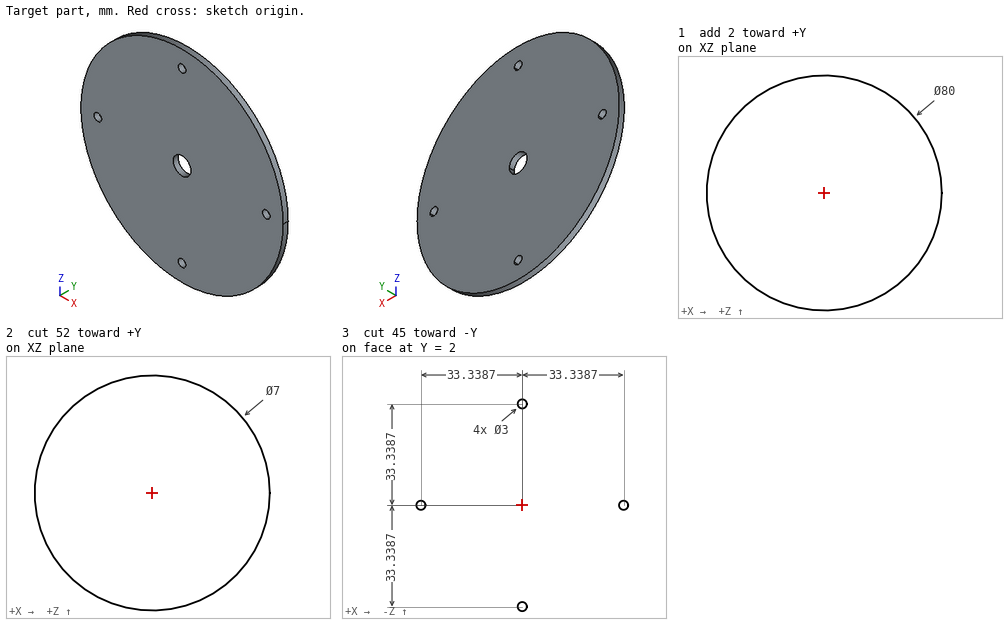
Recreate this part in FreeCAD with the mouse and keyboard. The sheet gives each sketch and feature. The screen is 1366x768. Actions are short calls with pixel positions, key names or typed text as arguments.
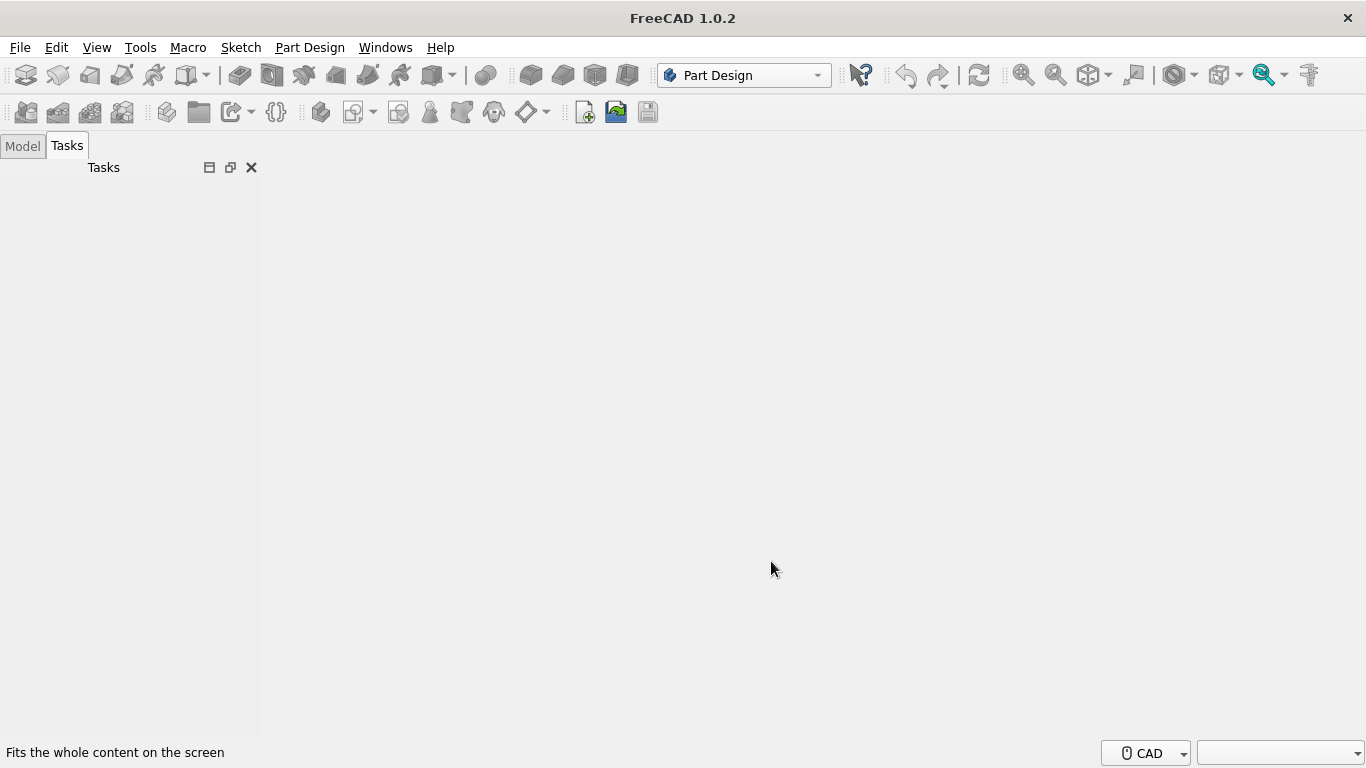
key(ctrl+n)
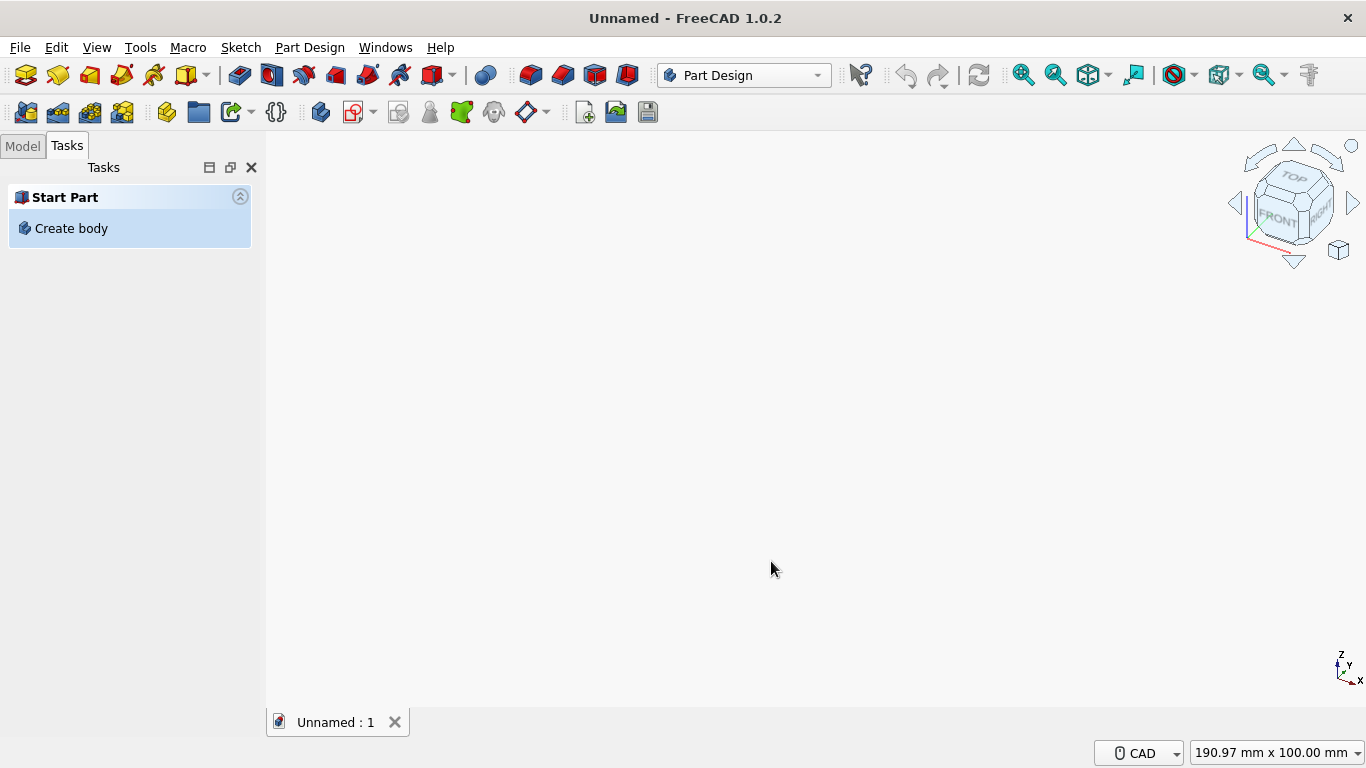
click(354, 112)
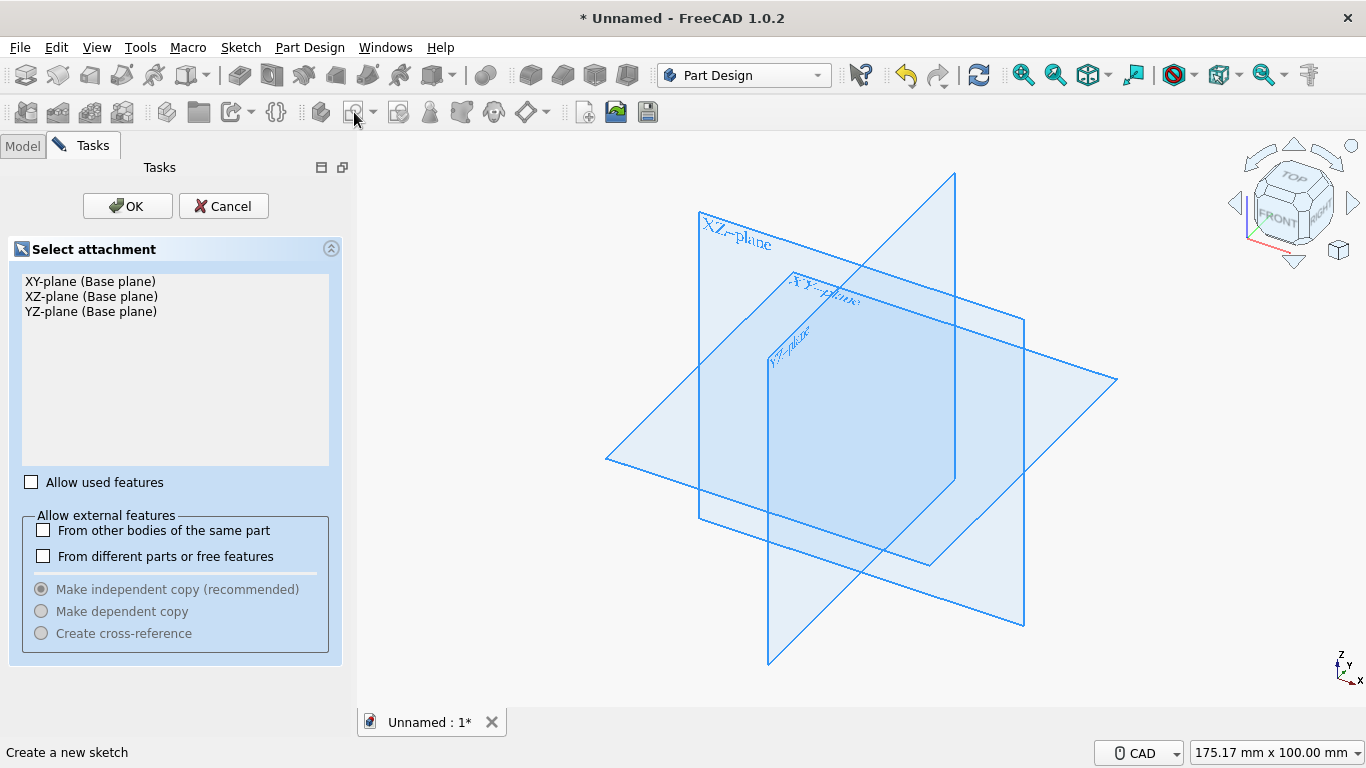
click(82, 296)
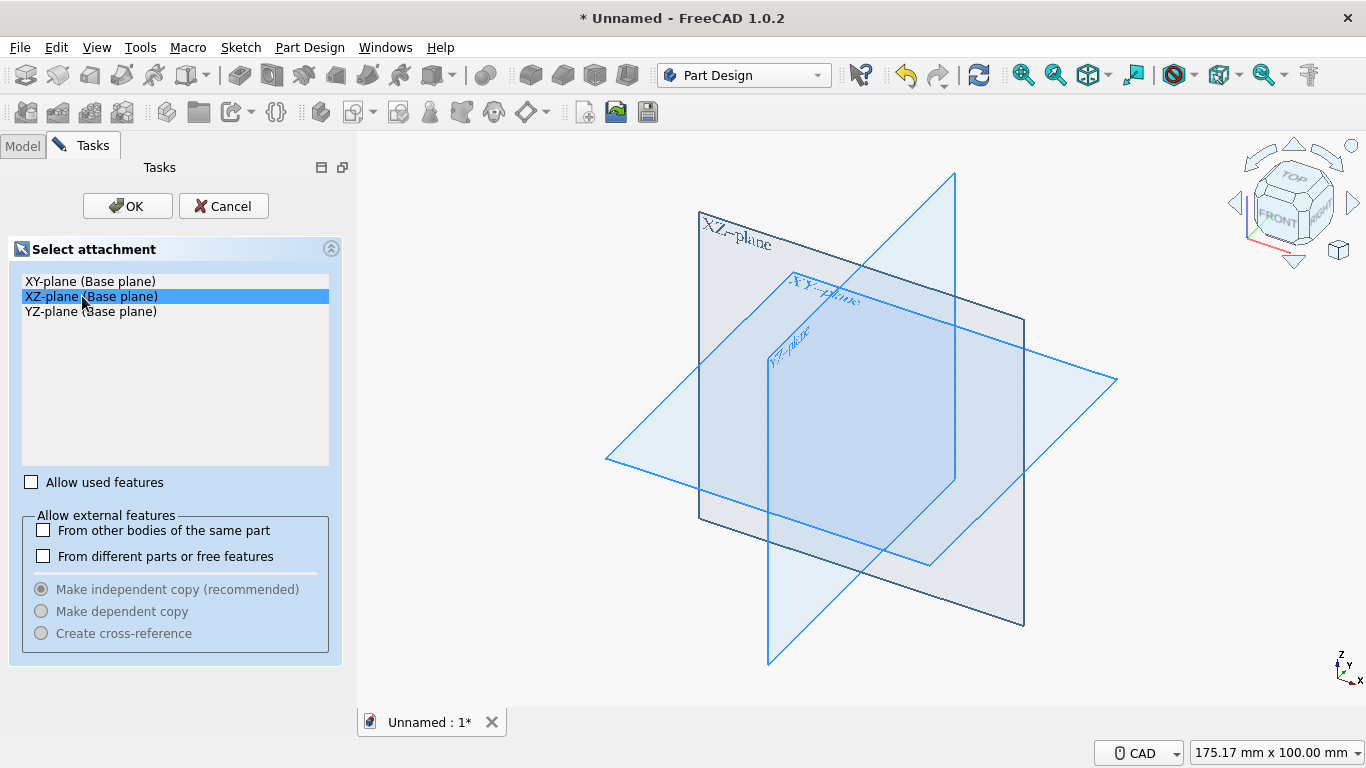
click(128, 206)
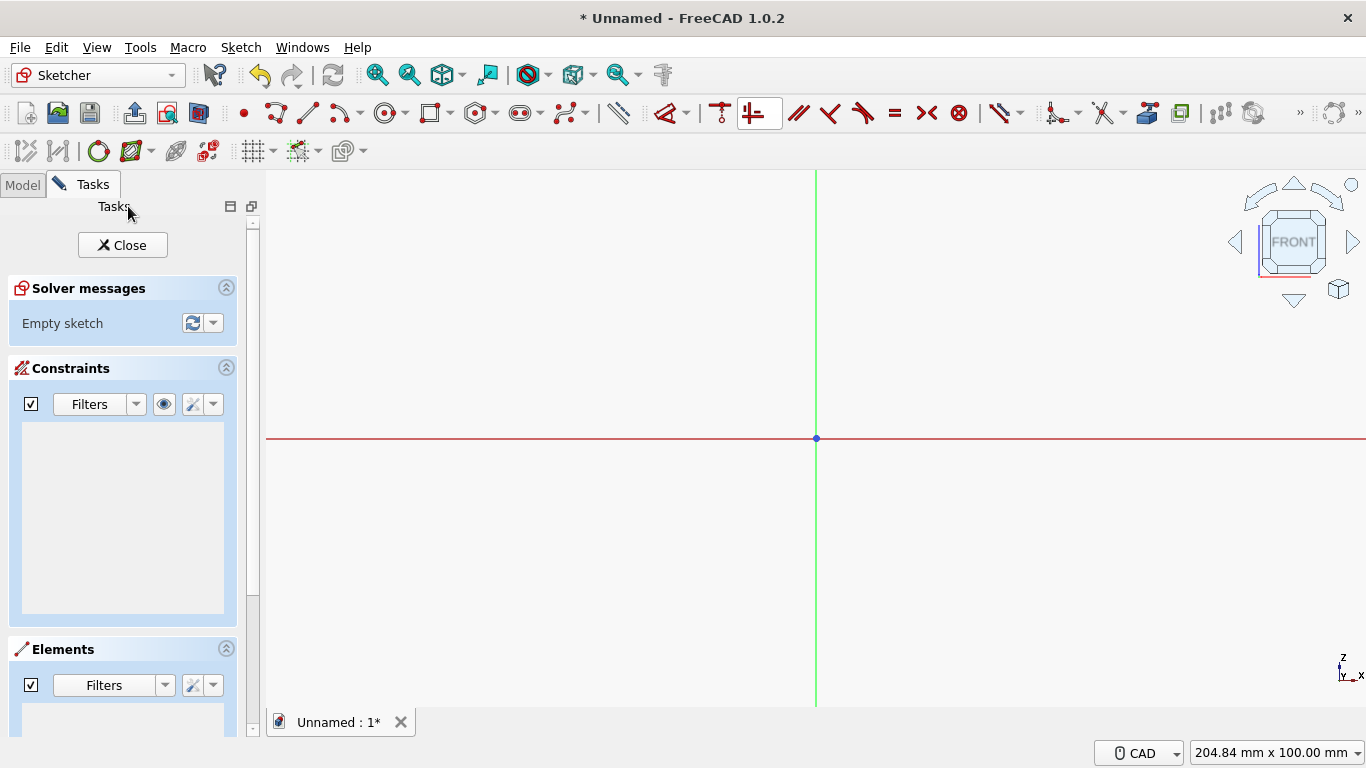
key(g)
key(c)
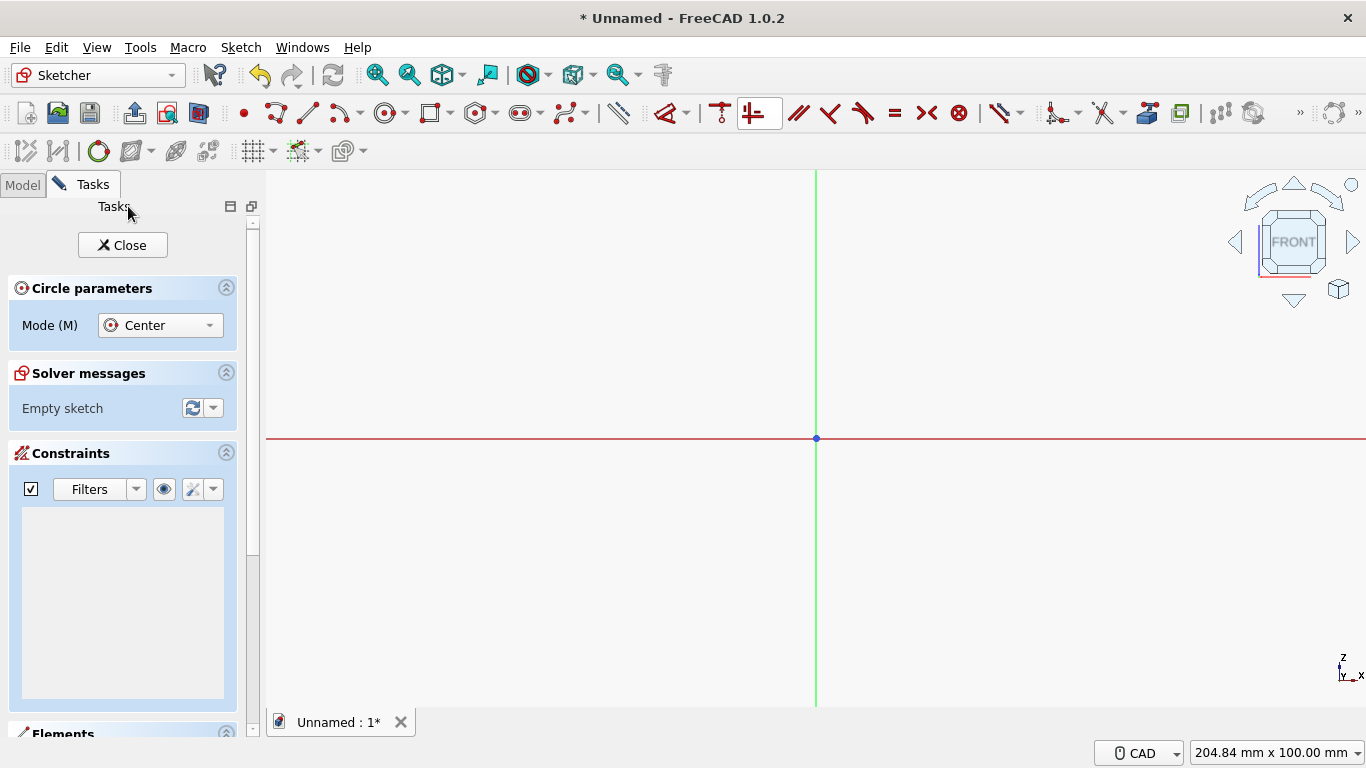
click(816, 438)
click(968, 287)
key(Escape)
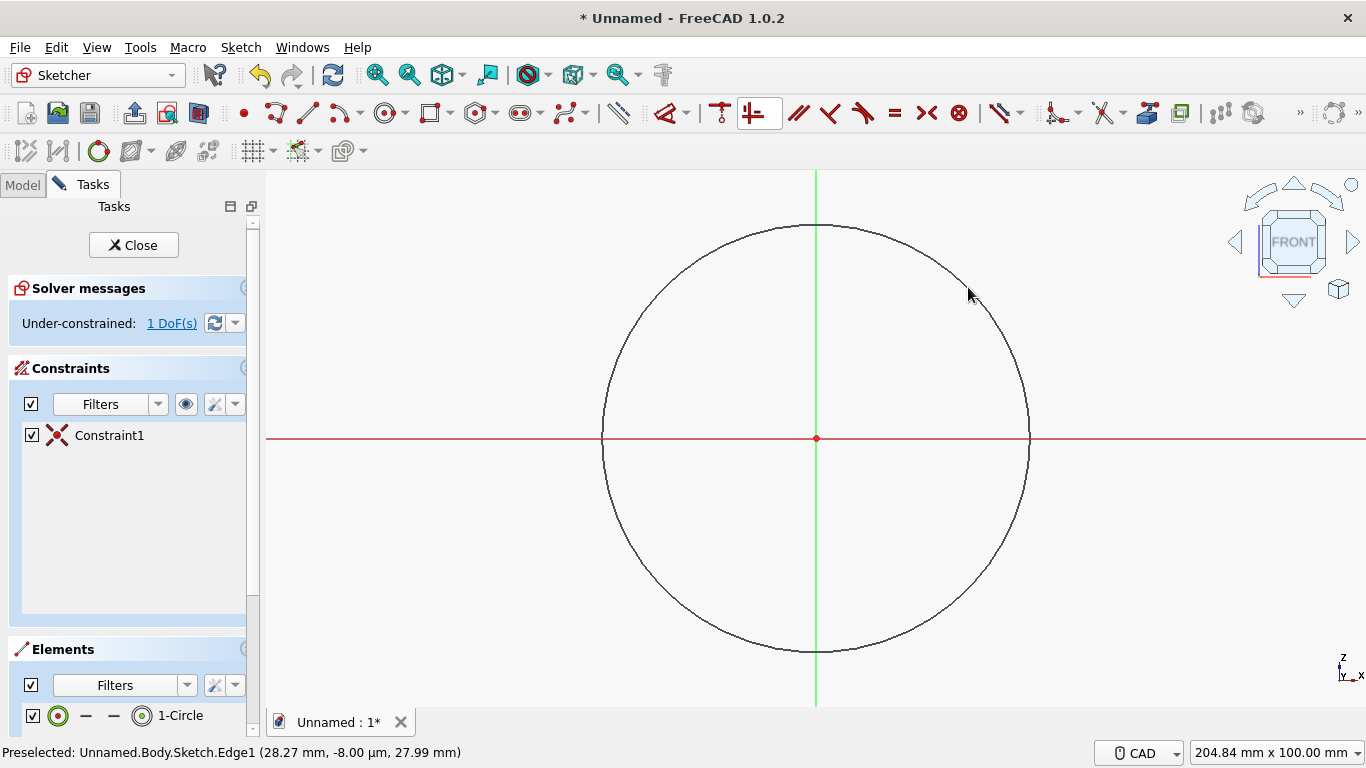
key(d)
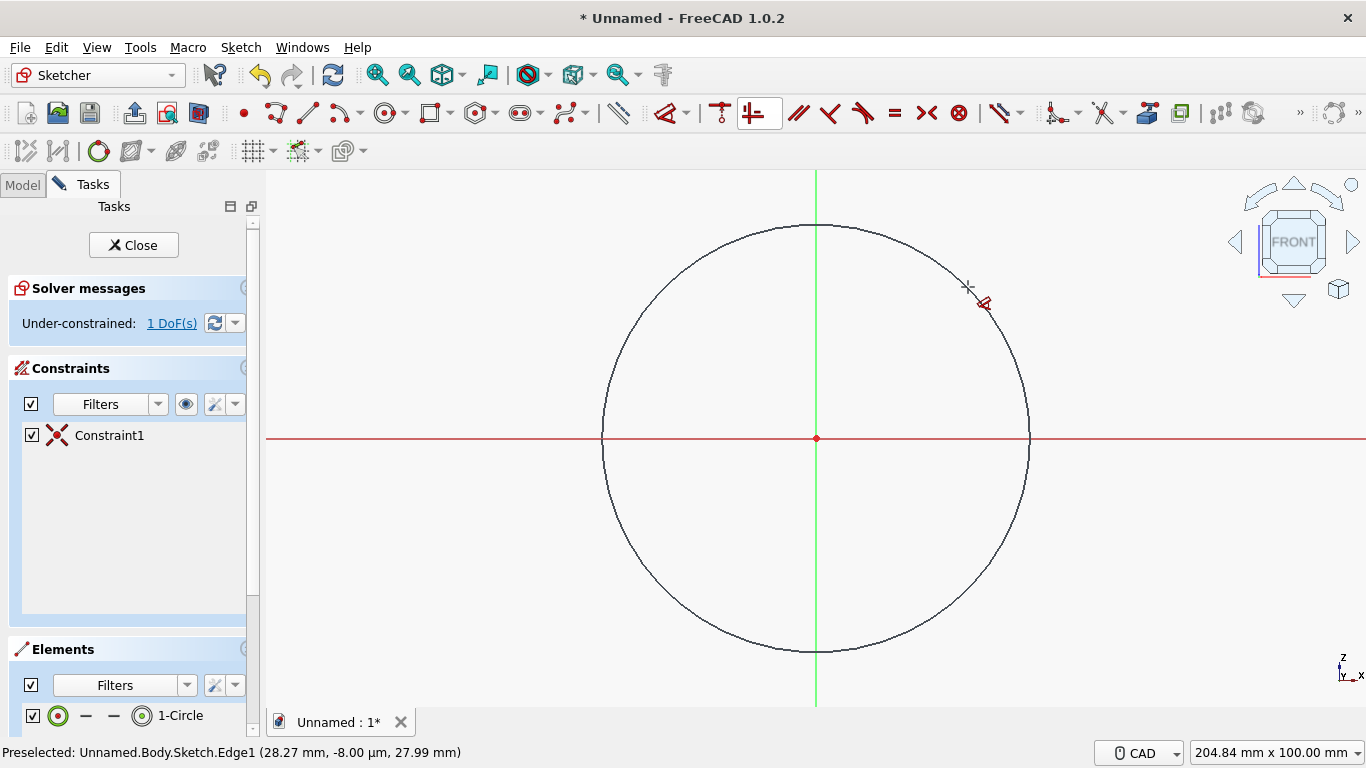
click(967, 287)
click(990, 264)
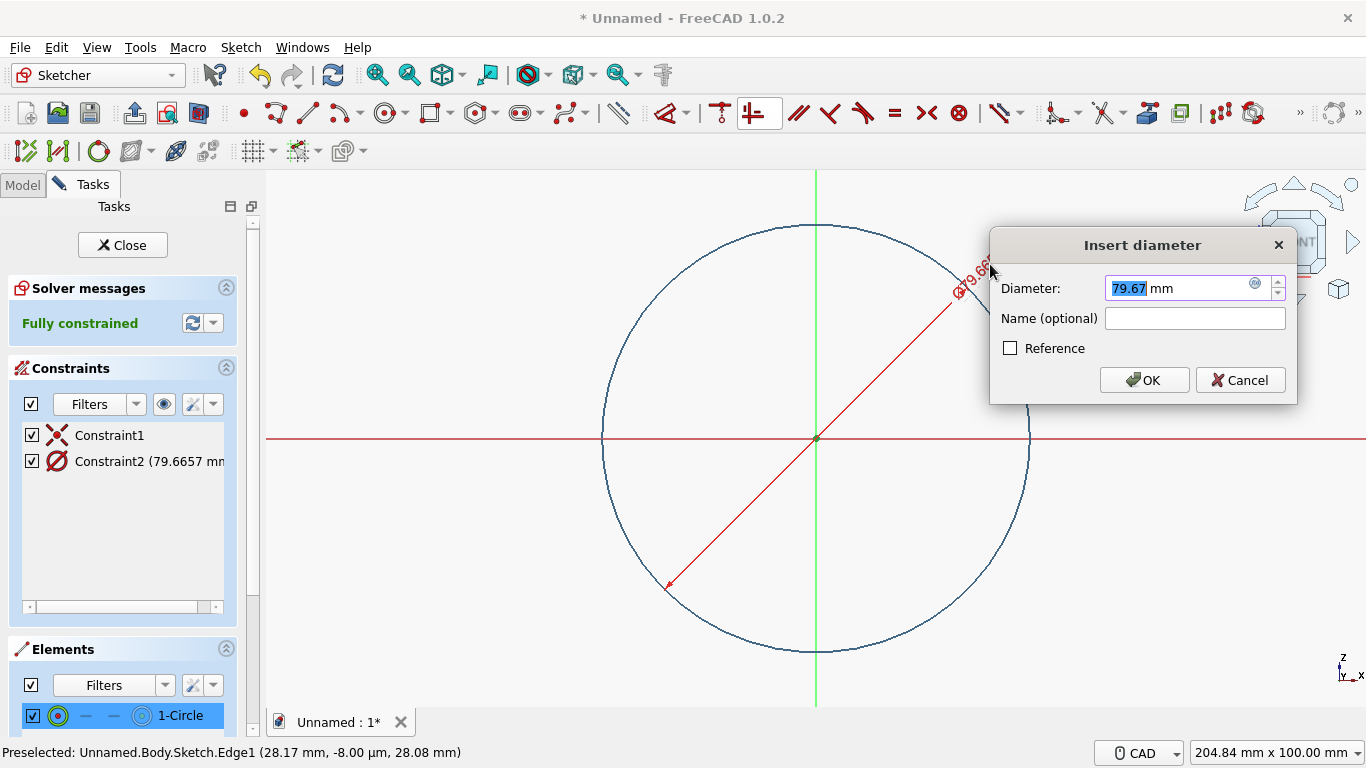
text(80)
key(Return)
key(Escape)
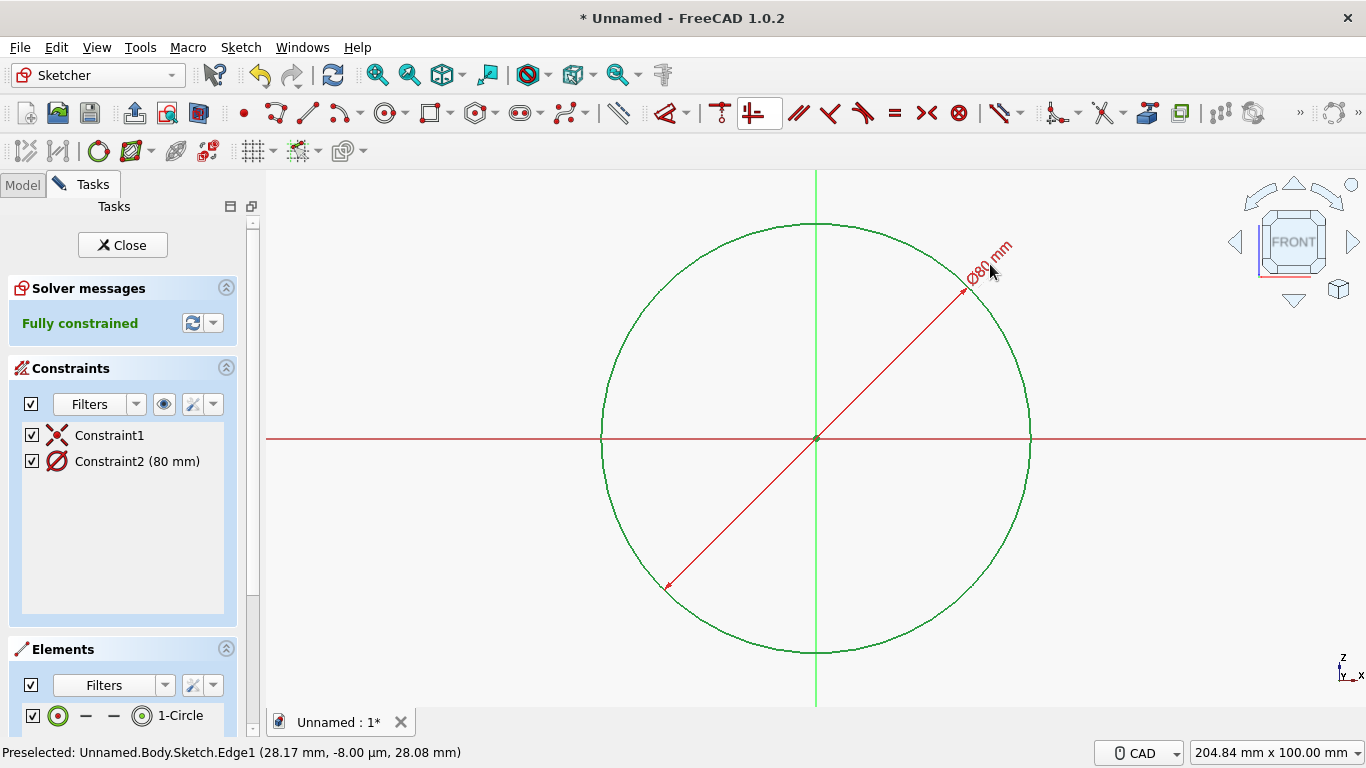
click(123, 245)